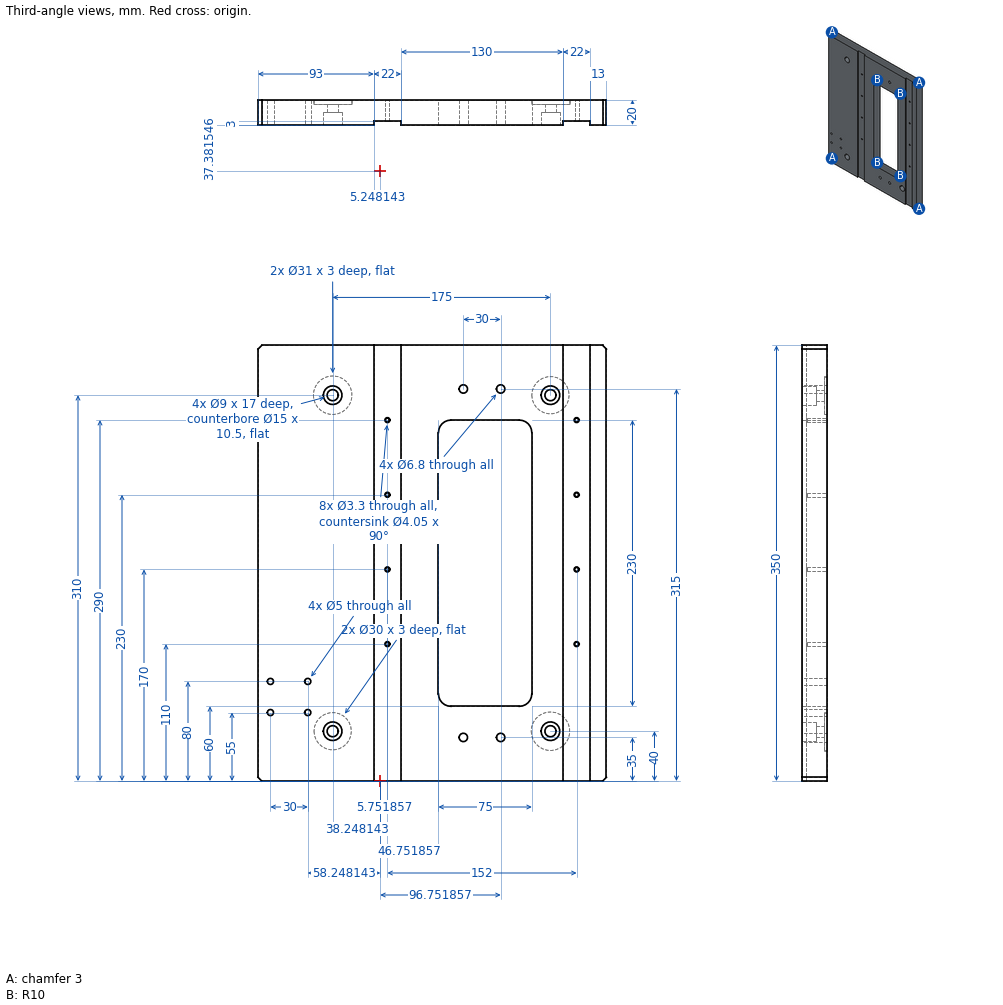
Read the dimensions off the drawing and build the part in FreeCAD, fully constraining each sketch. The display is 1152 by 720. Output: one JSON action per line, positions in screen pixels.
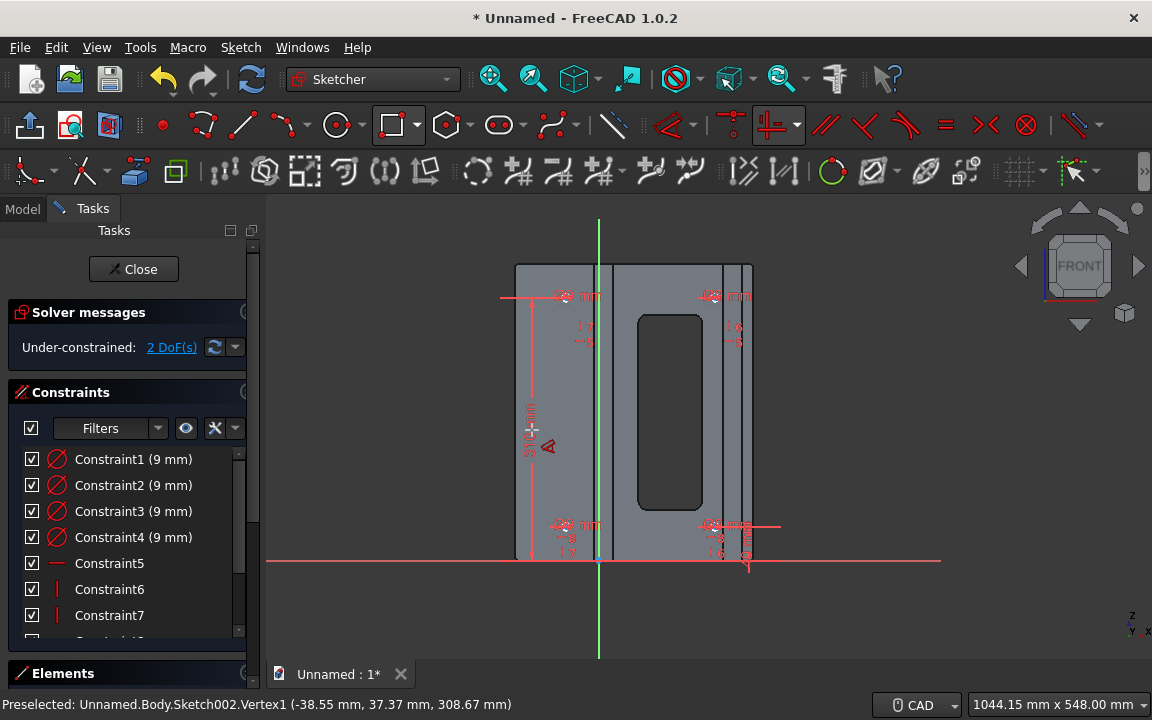
{"action": "left_click", "coordinate": [566, 298]}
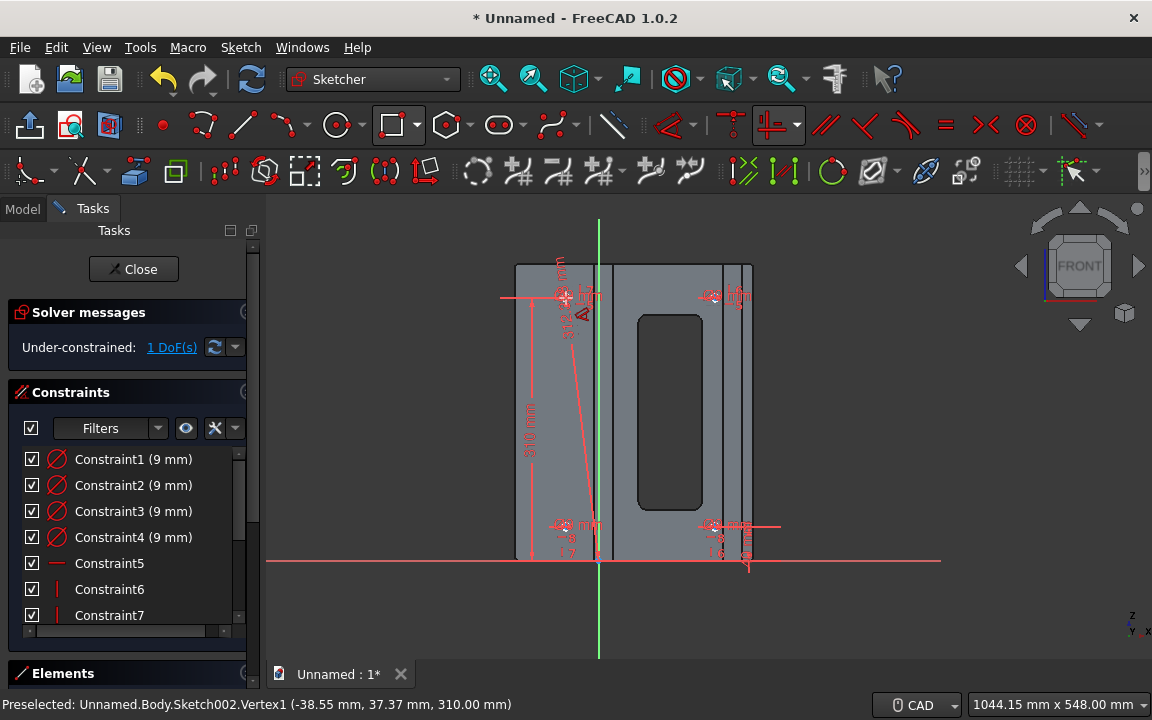
{"action": "left_click", "coordinate": [715, 298]}
{"action": "left_click", "coordinate": [641, 264]}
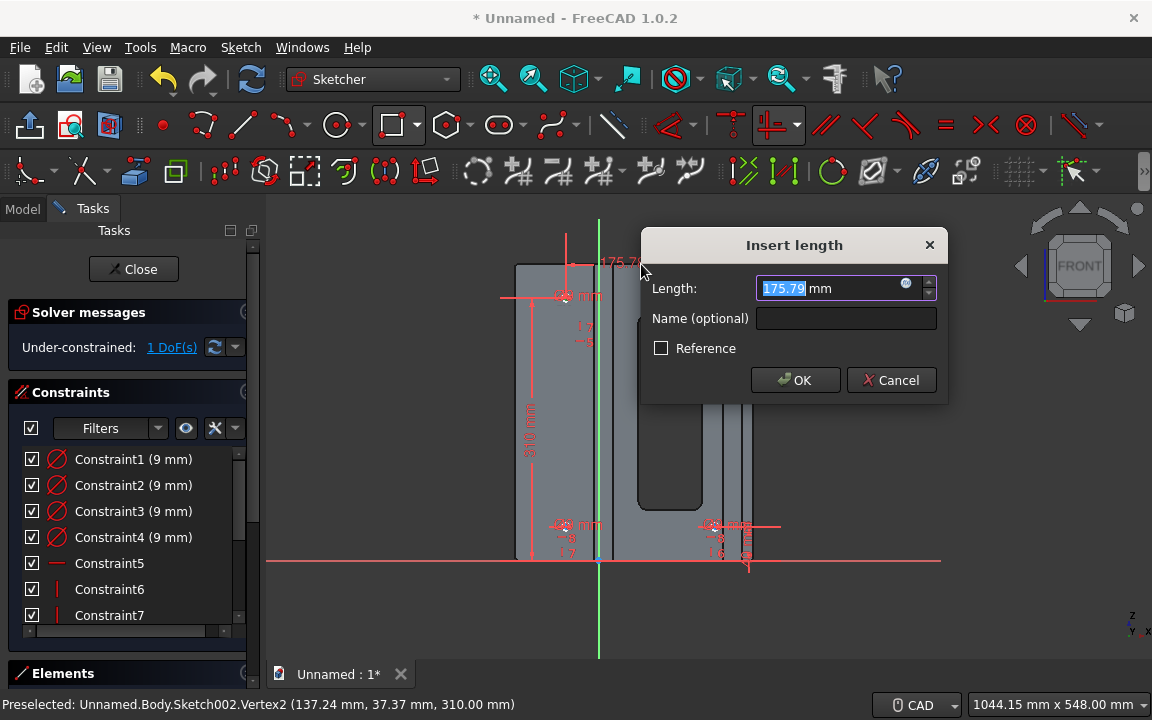
{"action": "type", "text": "175"}
{"action": "key", "text": "Return"}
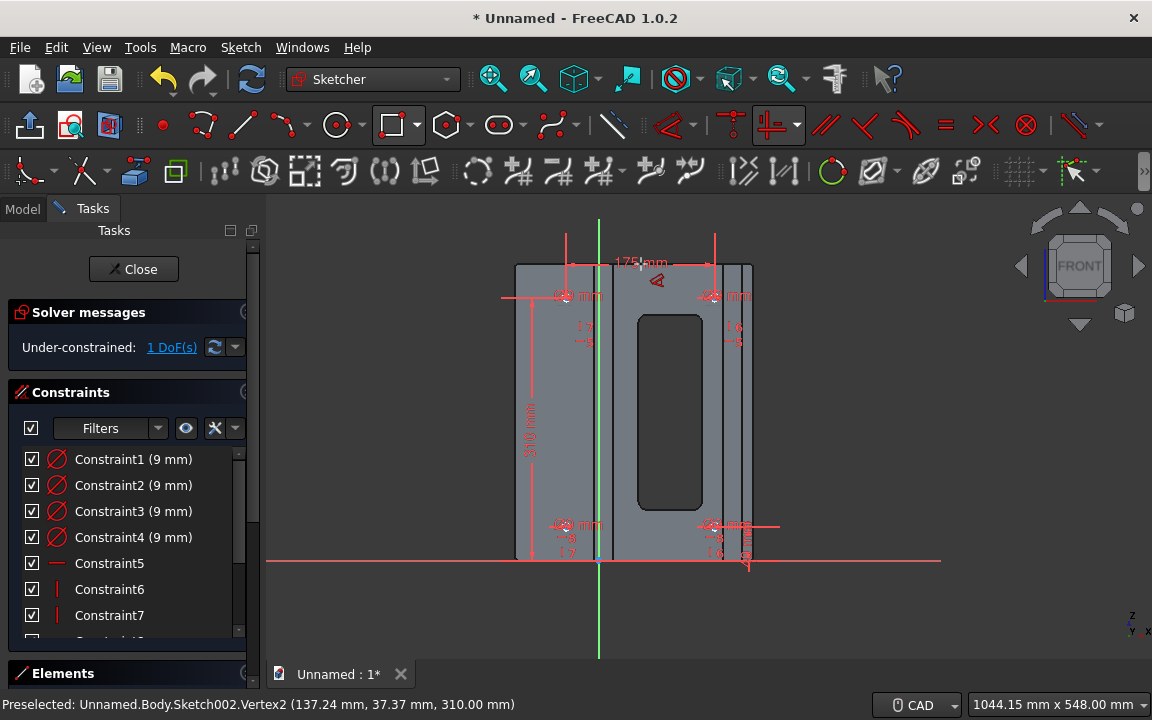
{"action": "scroll", "coordinate": [566, 298], "scroll_direction": "up", "scroll_amount": 2}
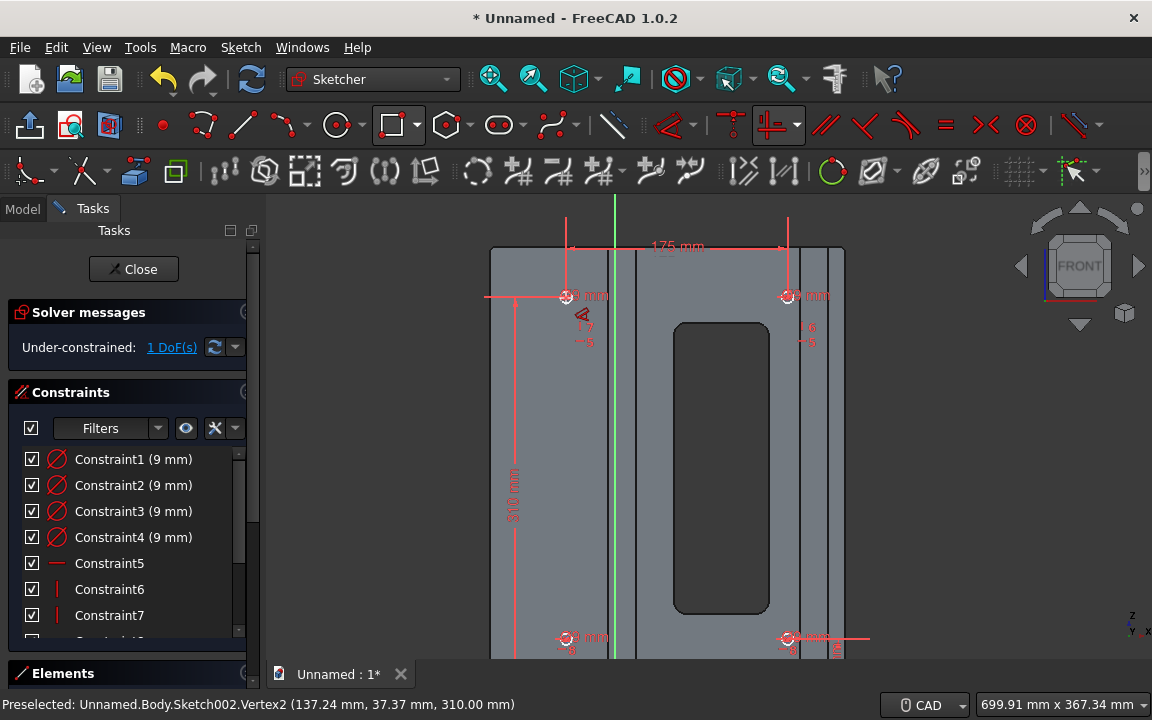
{"action": "left_click", "coordinate": [566, 297]}
{"action": "left_click", "coordinate": [590, 263]}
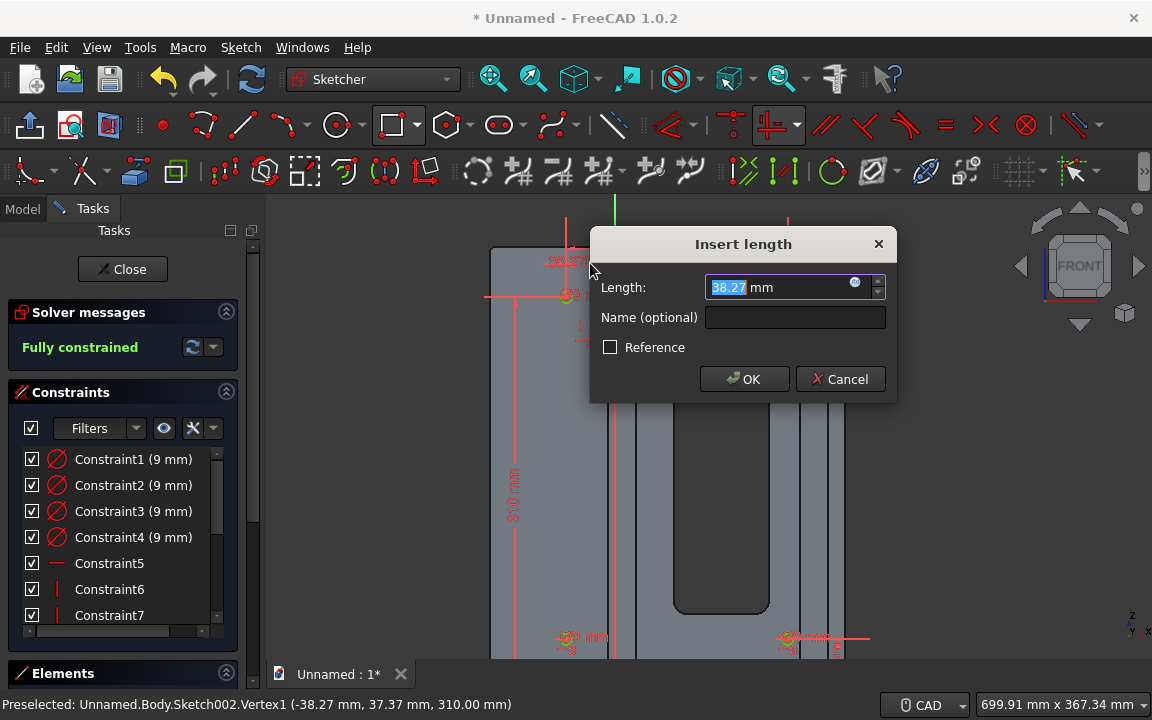
{"action": "type", "text": "38.248143"}
{"action": "key", "text": "Return"}
{"action": "key", "text": "Escape"}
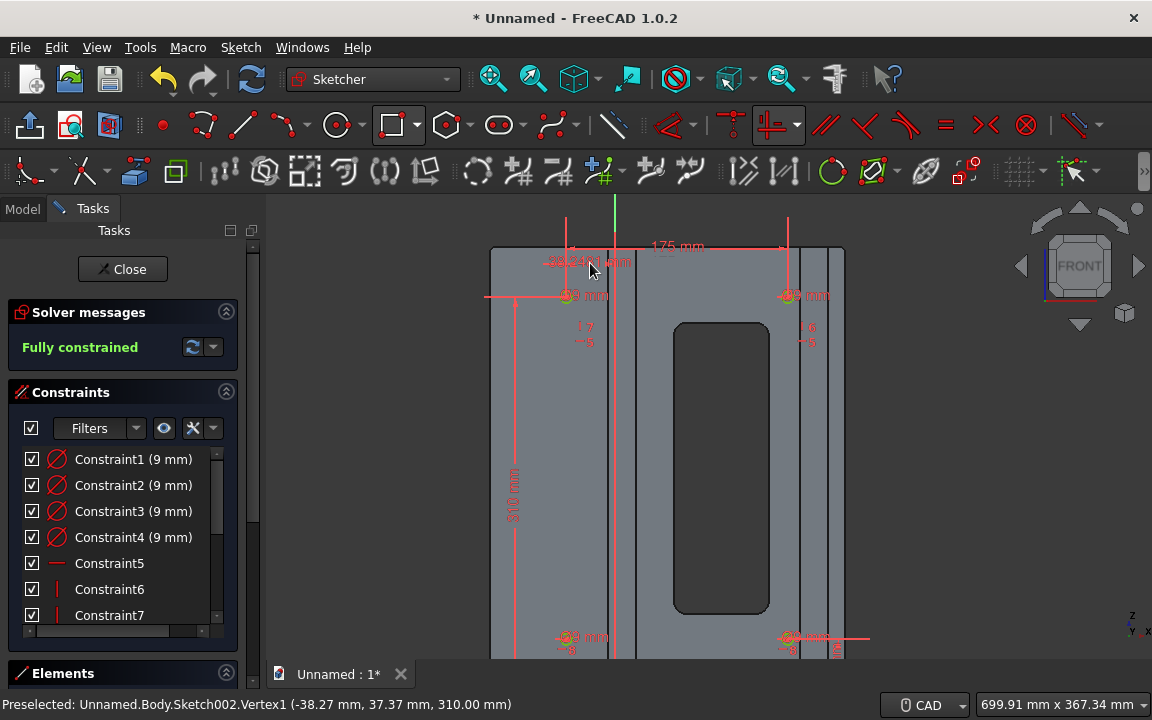
{"action": "left_click", "coordinate": [123, 269]}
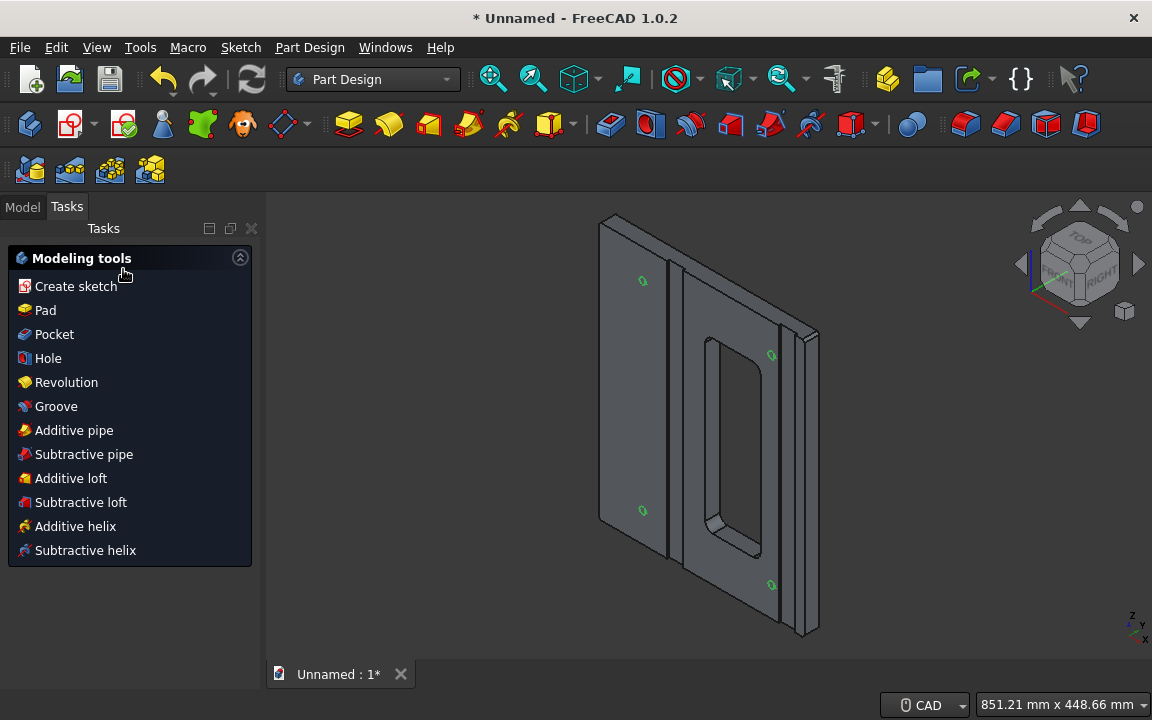
{"action": "left_click", "coordinate": [652, 124]}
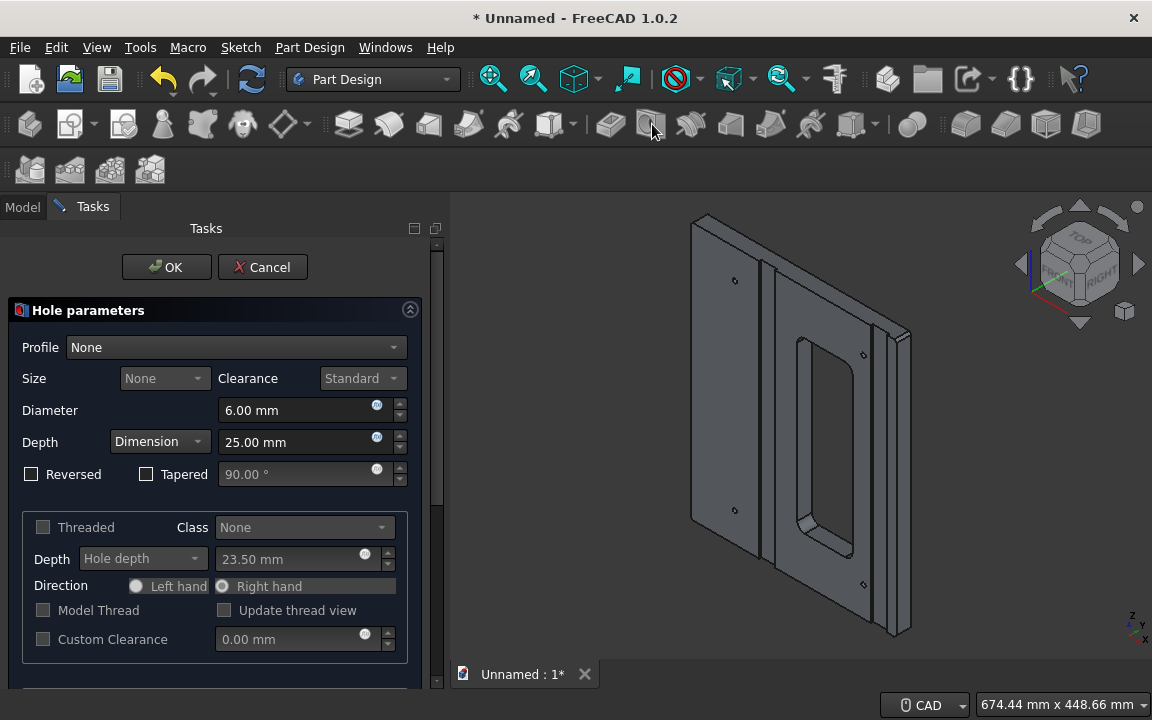
{"action": "triple_click", "coordinate": [305, 410]}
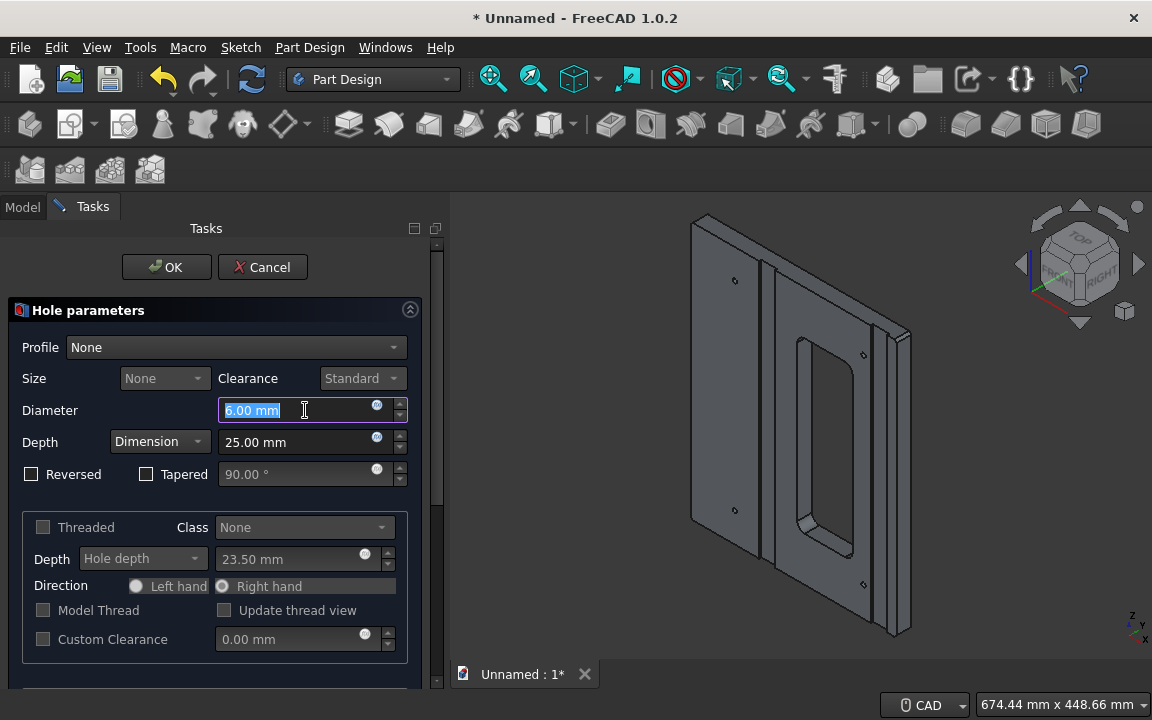
{"action": "type", "text": "9"}
{"action": "key", "text": "Tab"}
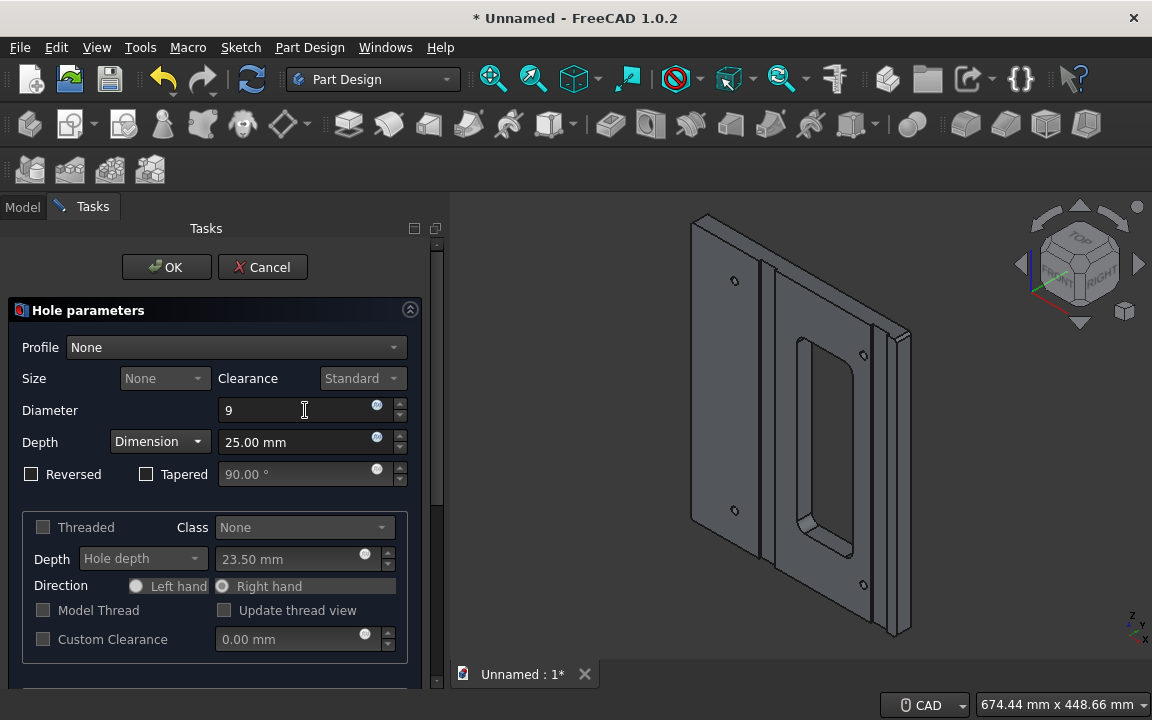
{"action": "triple_click", "coordinate": [305, 442]}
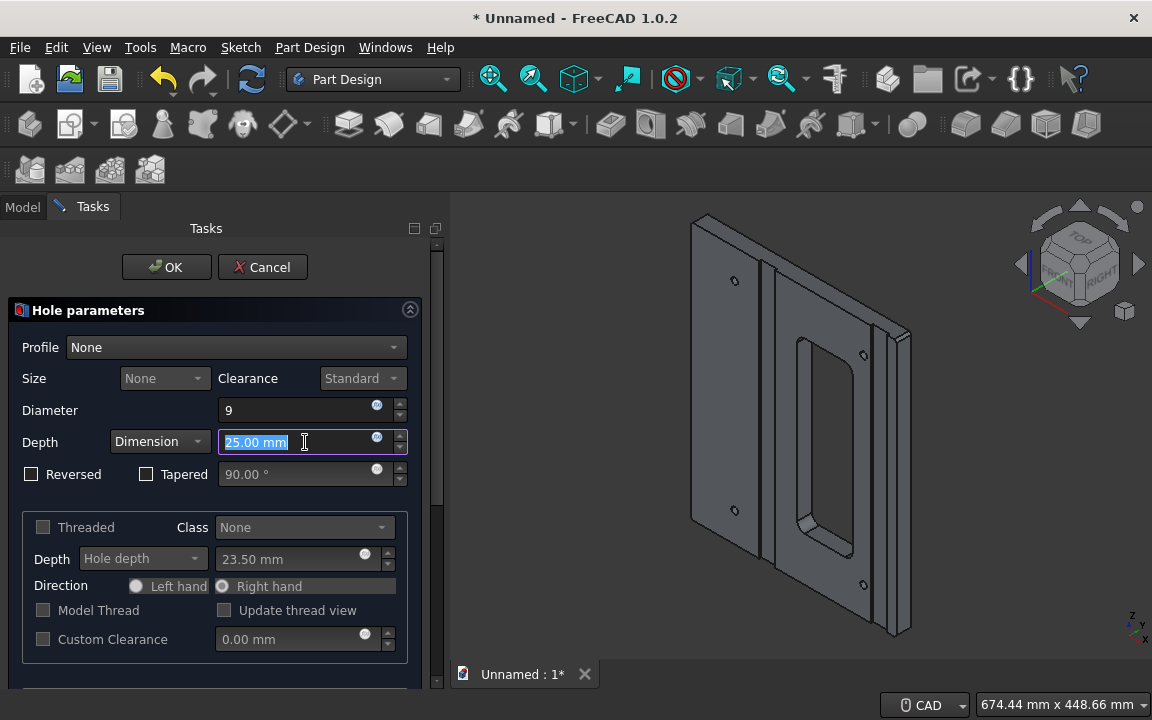
{"action": "type", "text": "17"}
{"action": "key", "text": "Tab"}